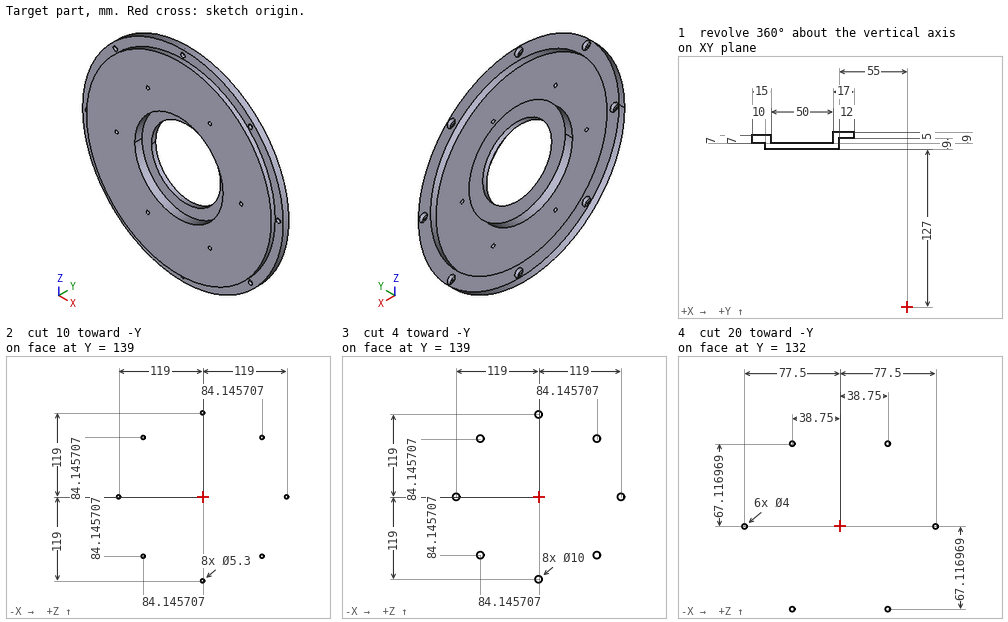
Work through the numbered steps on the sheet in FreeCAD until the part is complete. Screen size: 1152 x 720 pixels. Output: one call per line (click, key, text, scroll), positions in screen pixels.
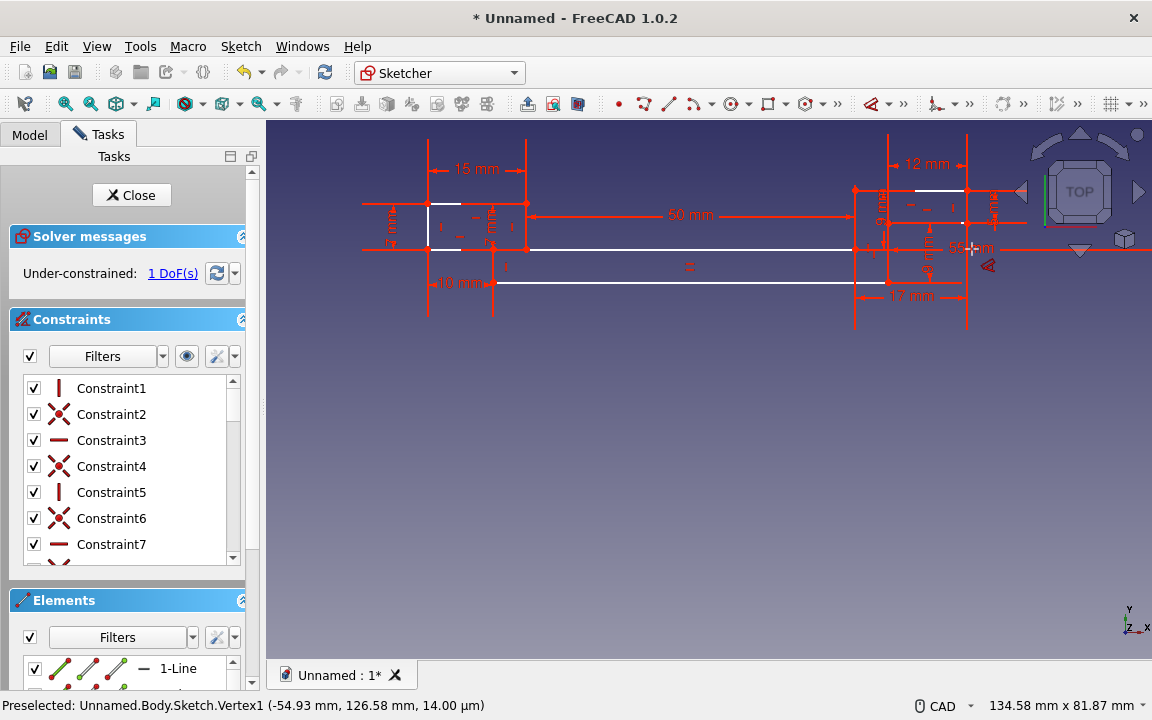
click(888, 283)
click(854, 457)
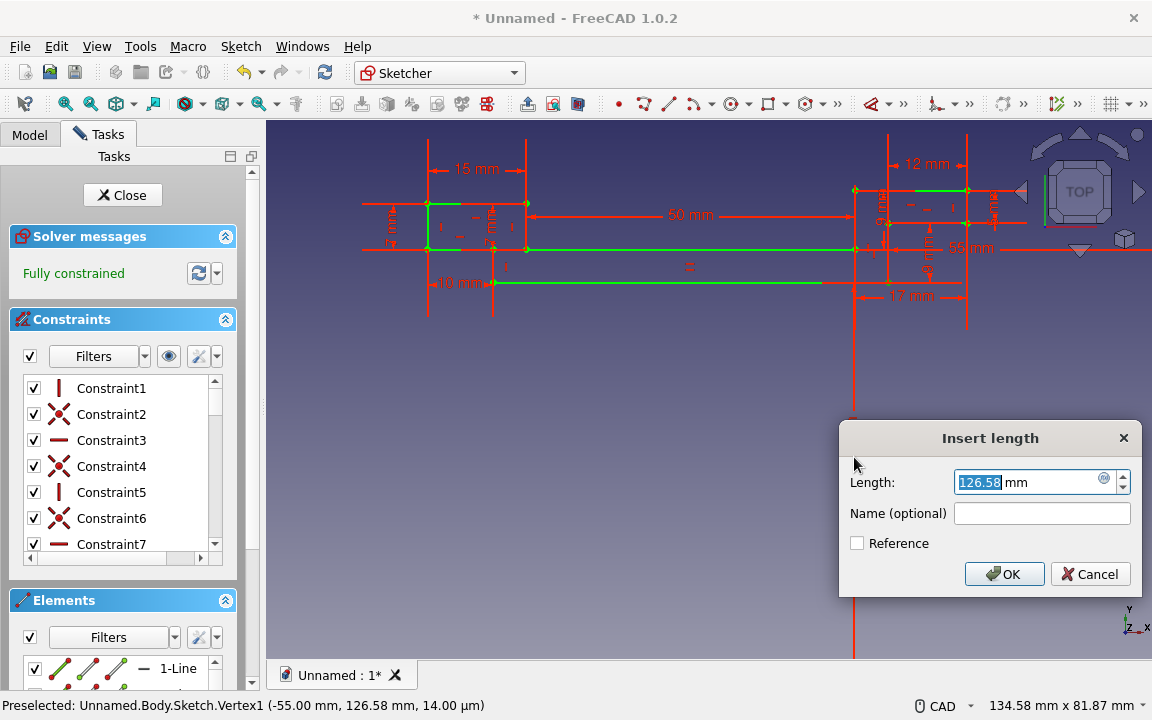
text(127)
key(Return)
key(Escape)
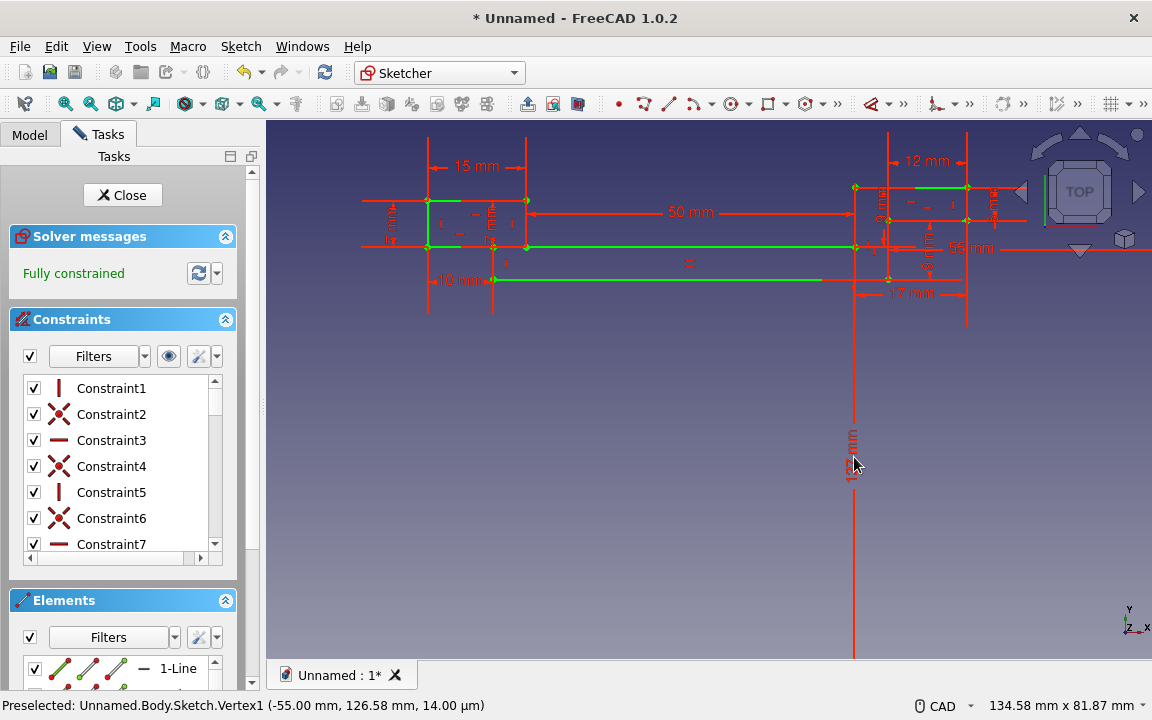
click(123, 195)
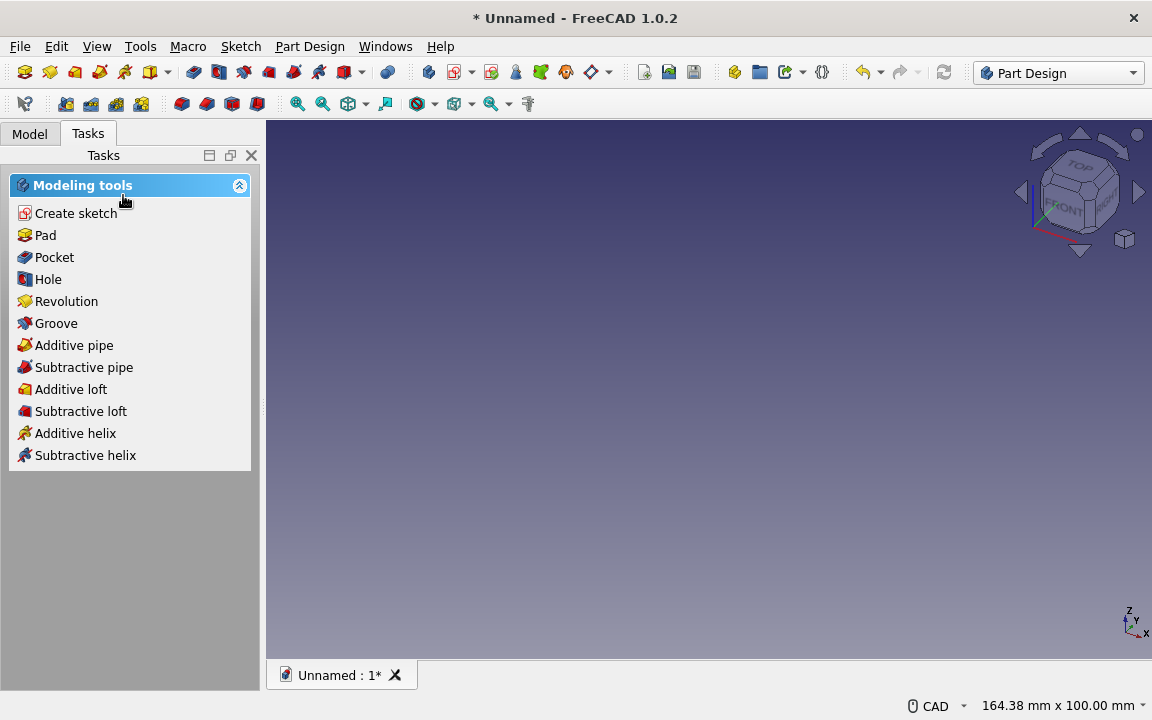
click(50, 72)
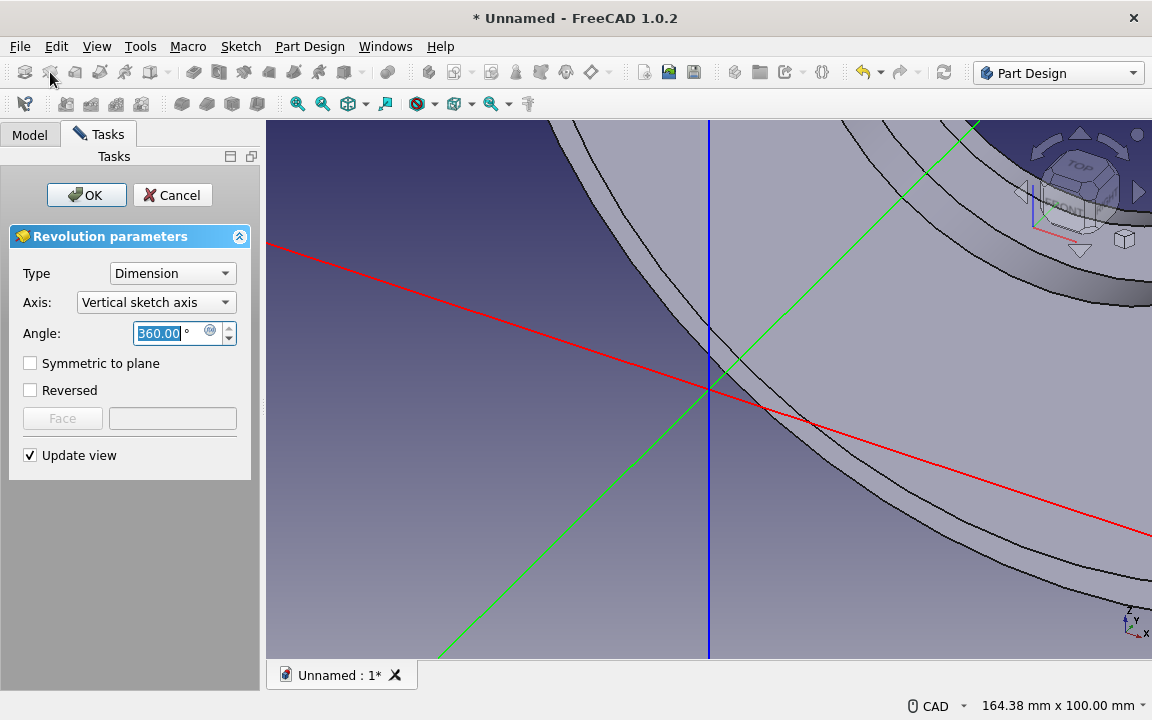
click(87, 195)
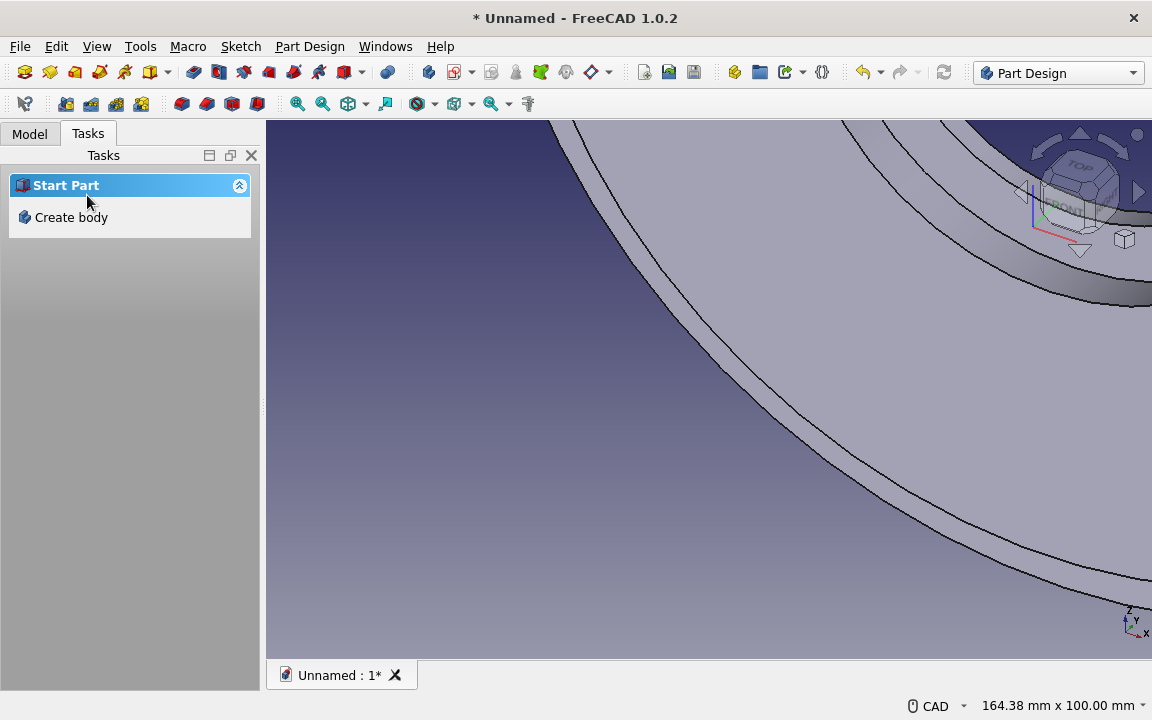
click(298, 104)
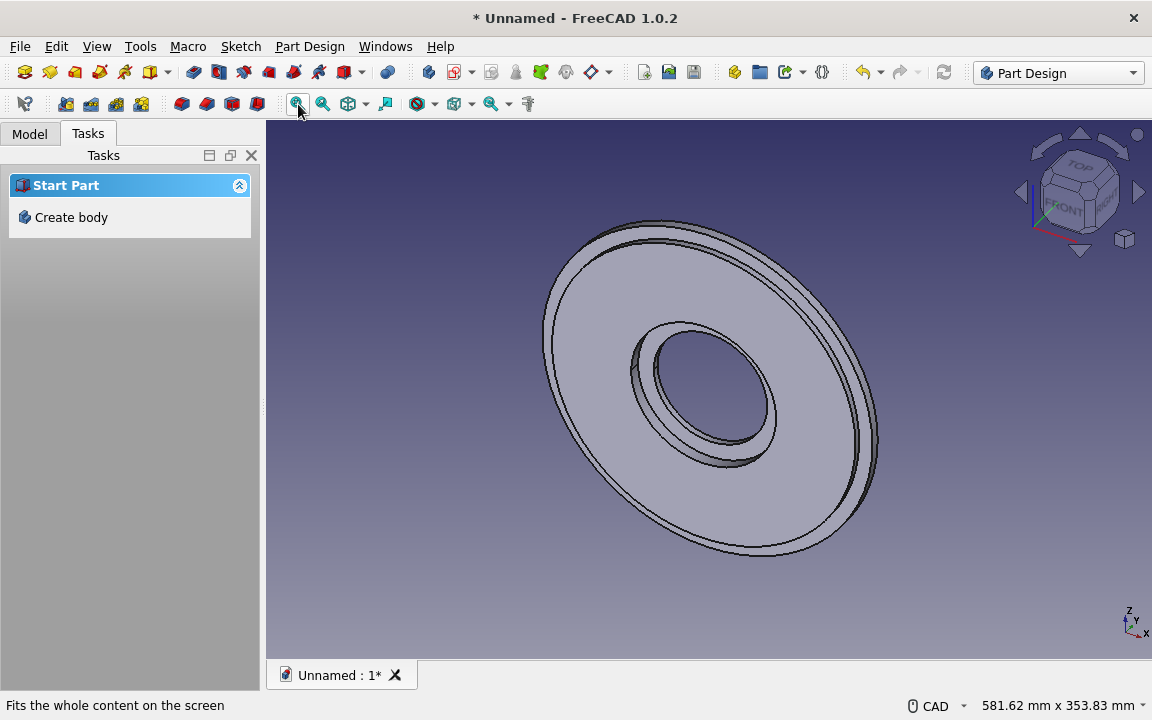
key(4)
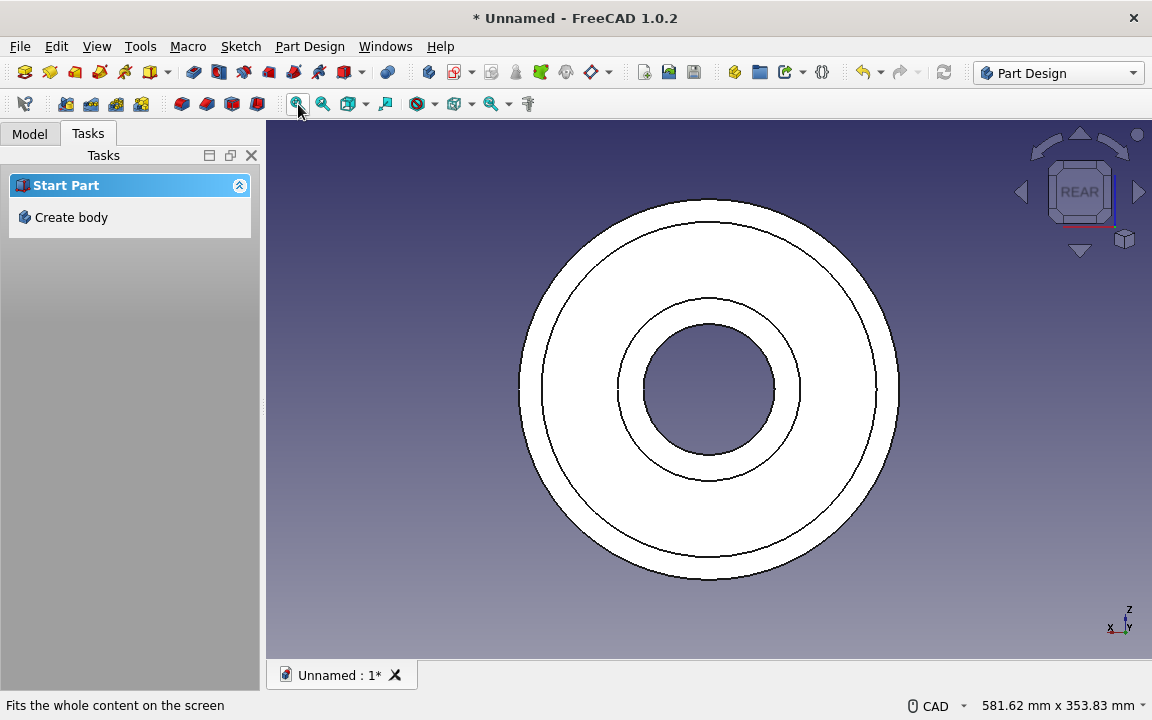
scroll(546, 334, up, 5)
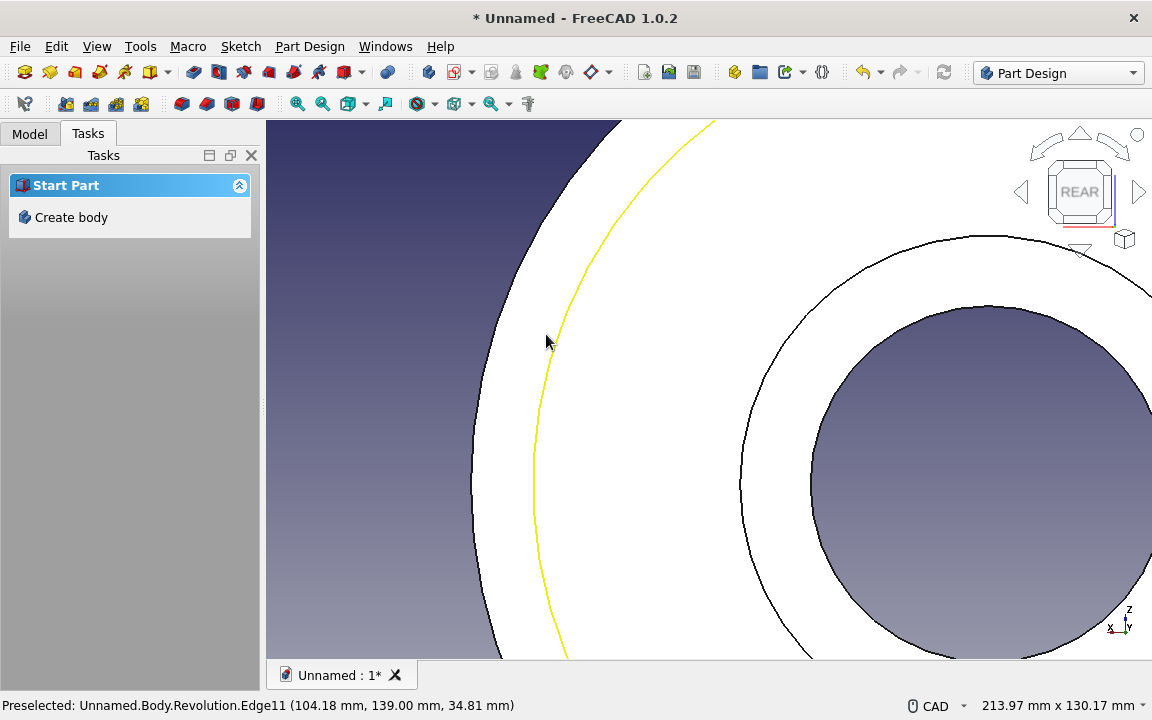
click(545, 335)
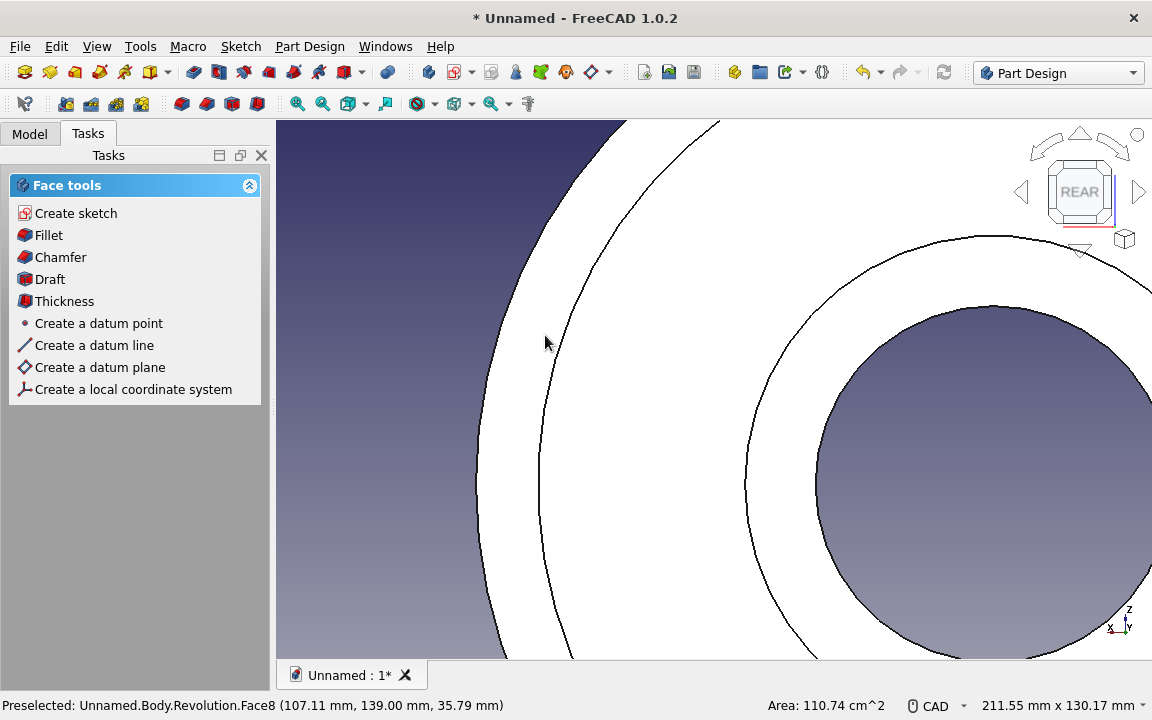
click(454, 72)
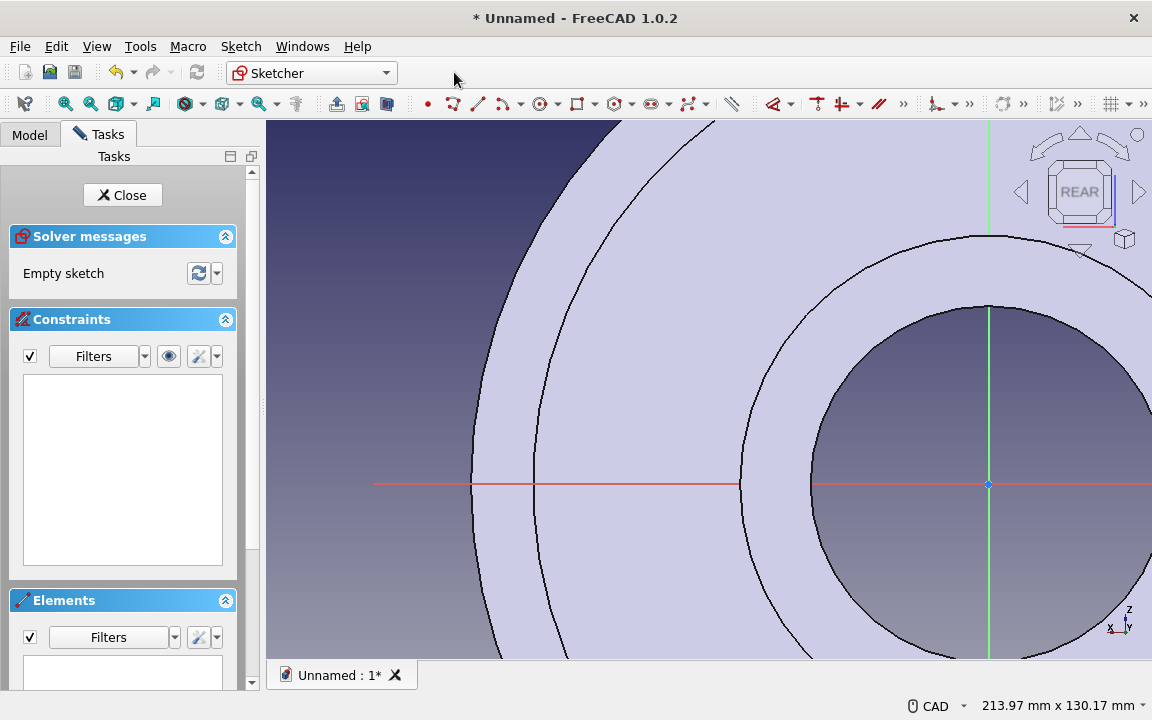
scroll(438, 334, down, 5)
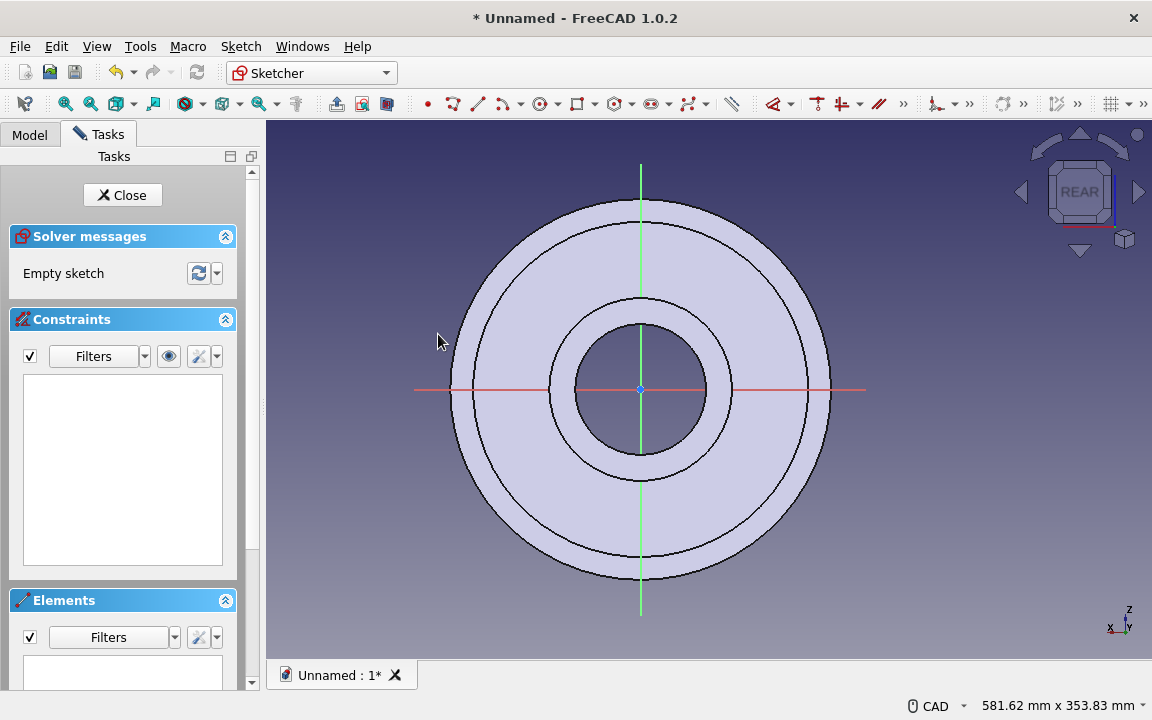
click(540, 104)